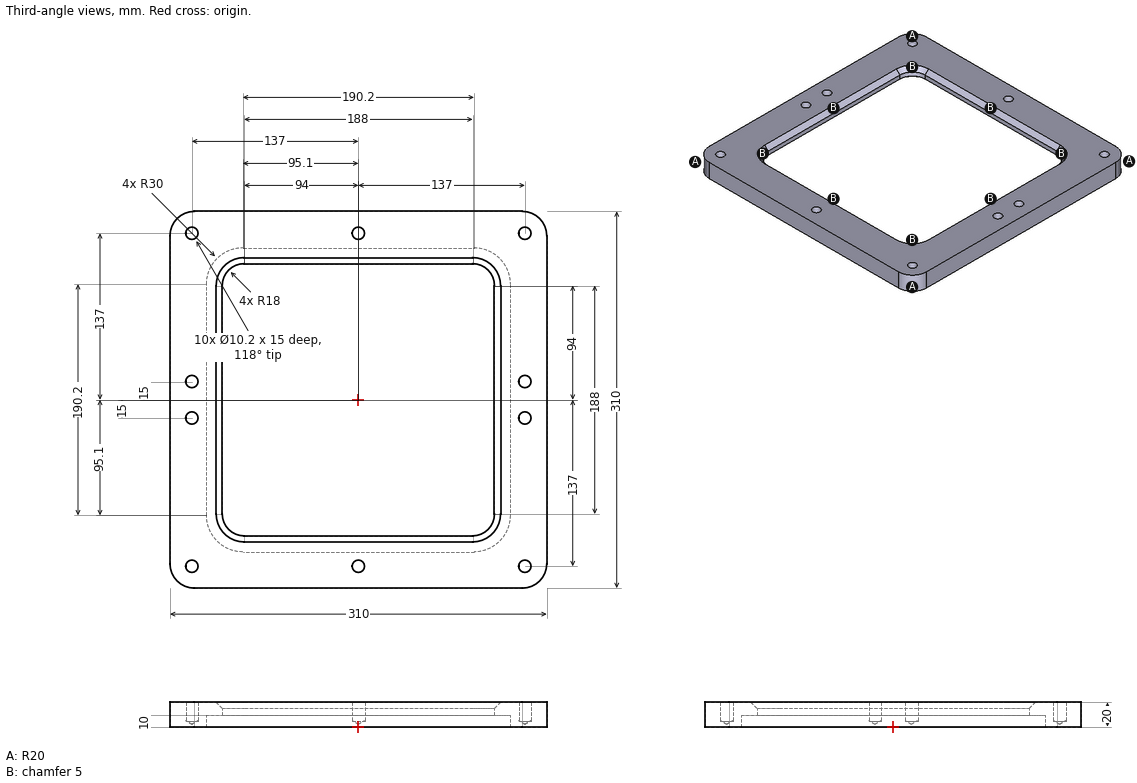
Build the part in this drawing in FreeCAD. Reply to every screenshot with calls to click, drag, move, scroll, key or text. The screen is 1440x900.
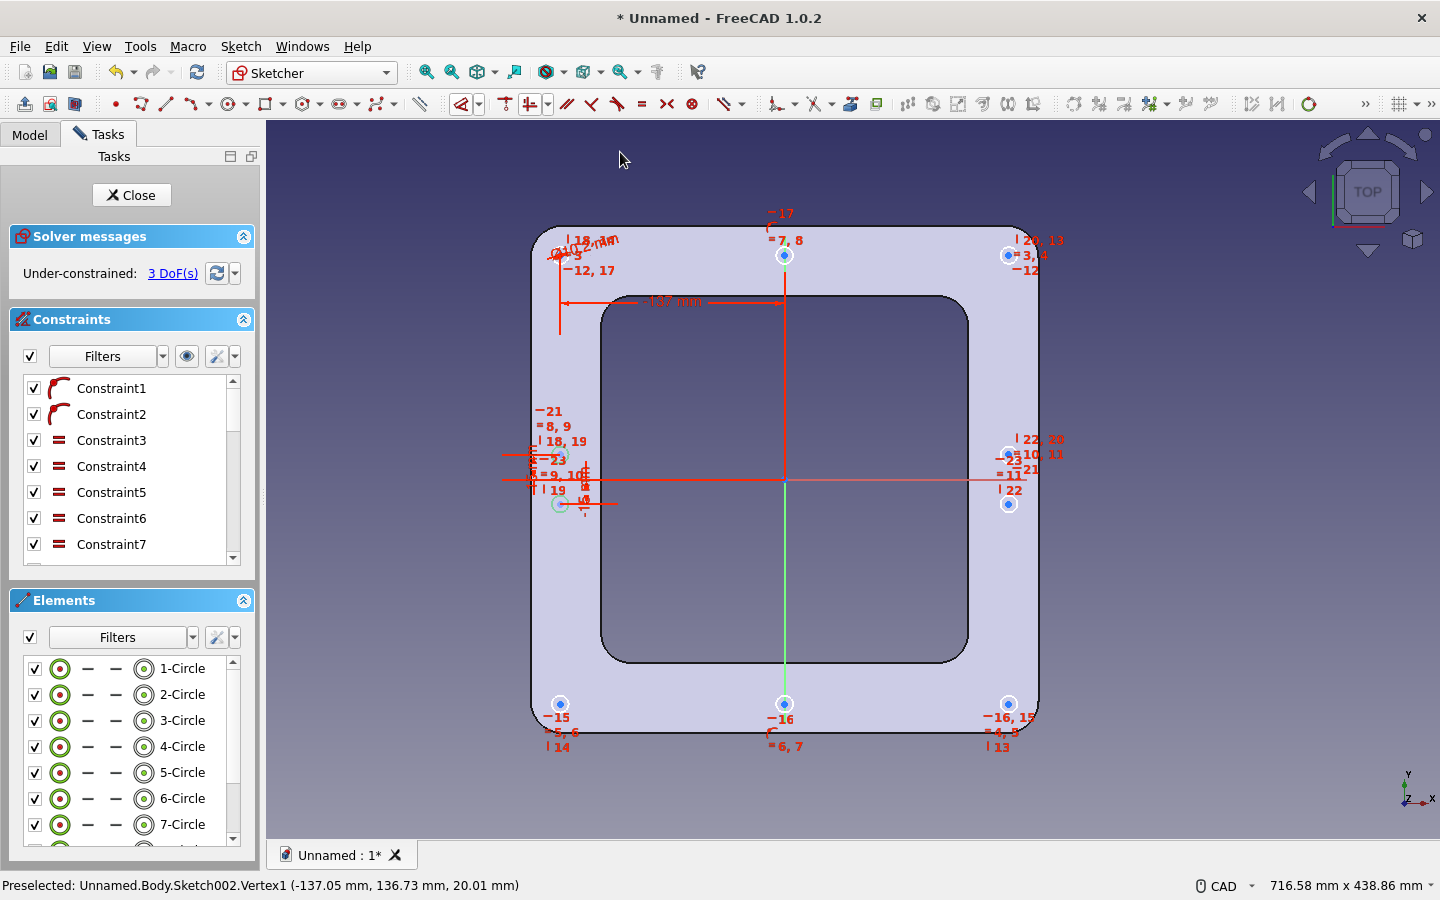
click(560, 255)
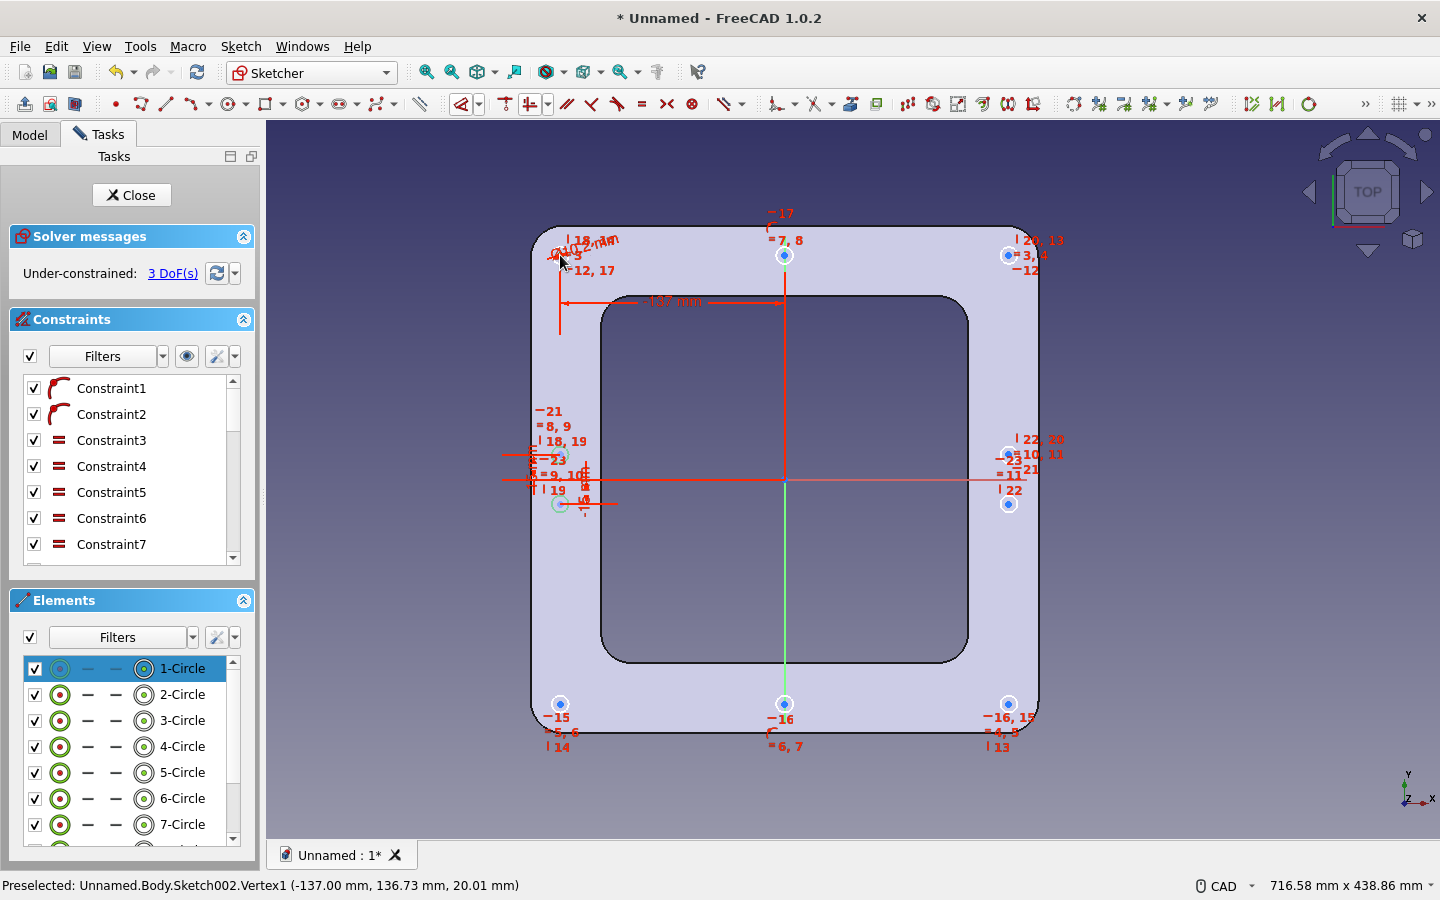
click(478, 104)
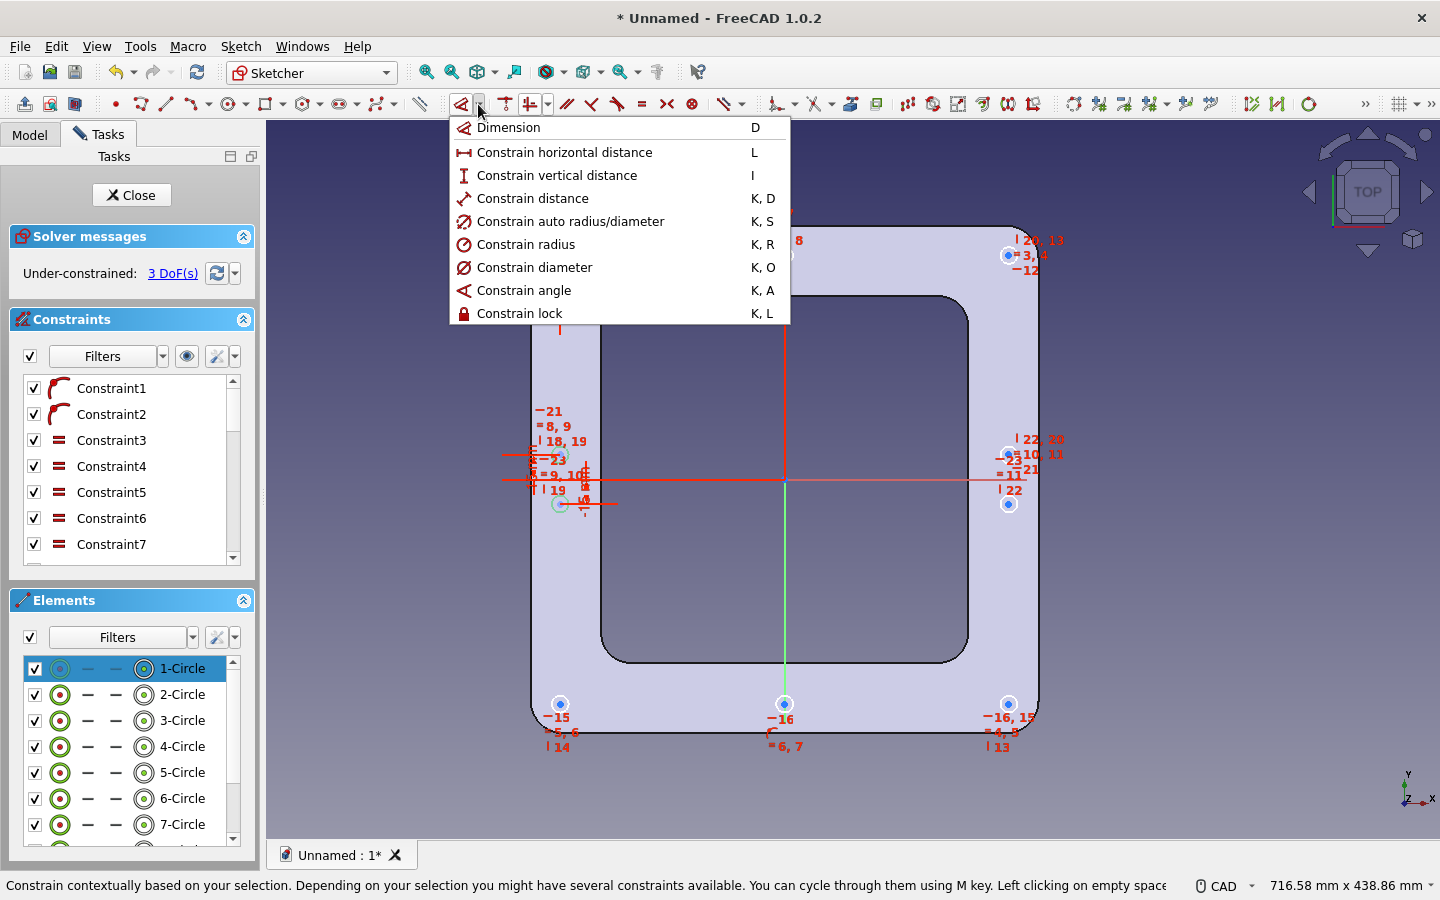
click(620, 176)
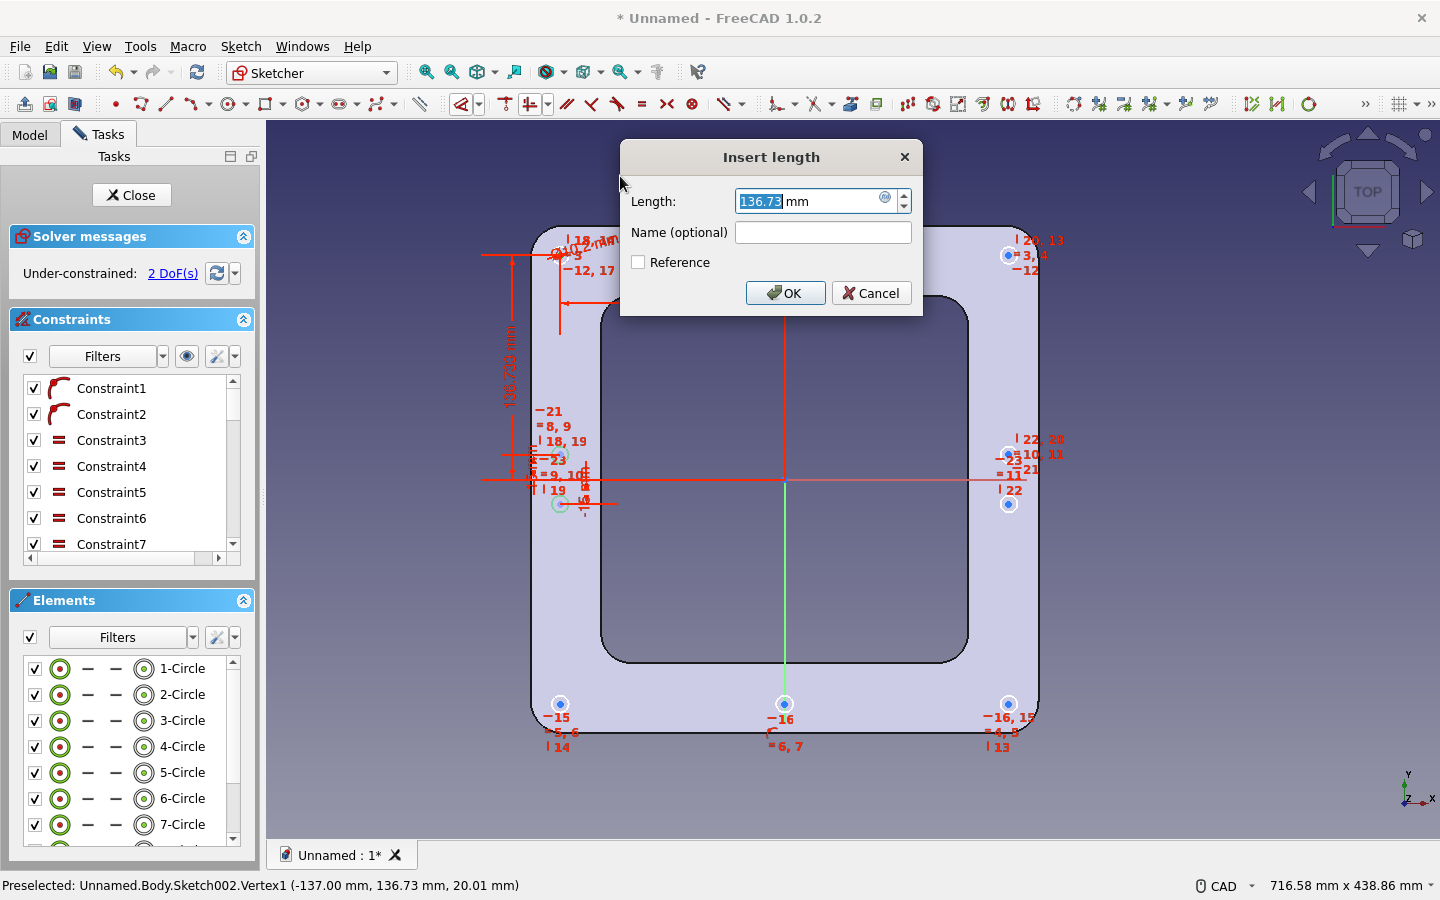
text(137)
key(Return)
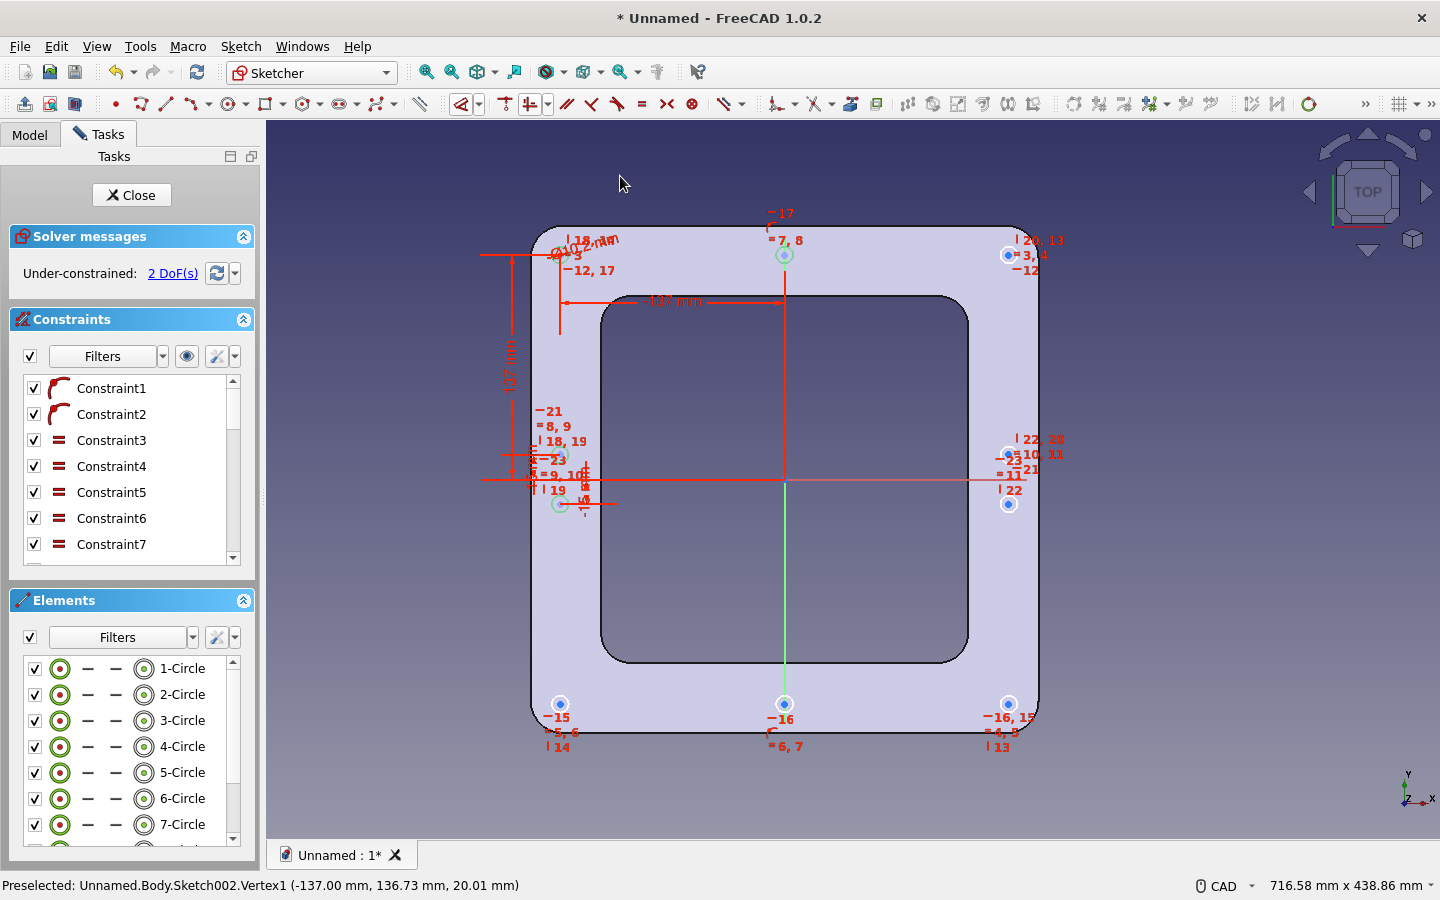
click(1009, 255)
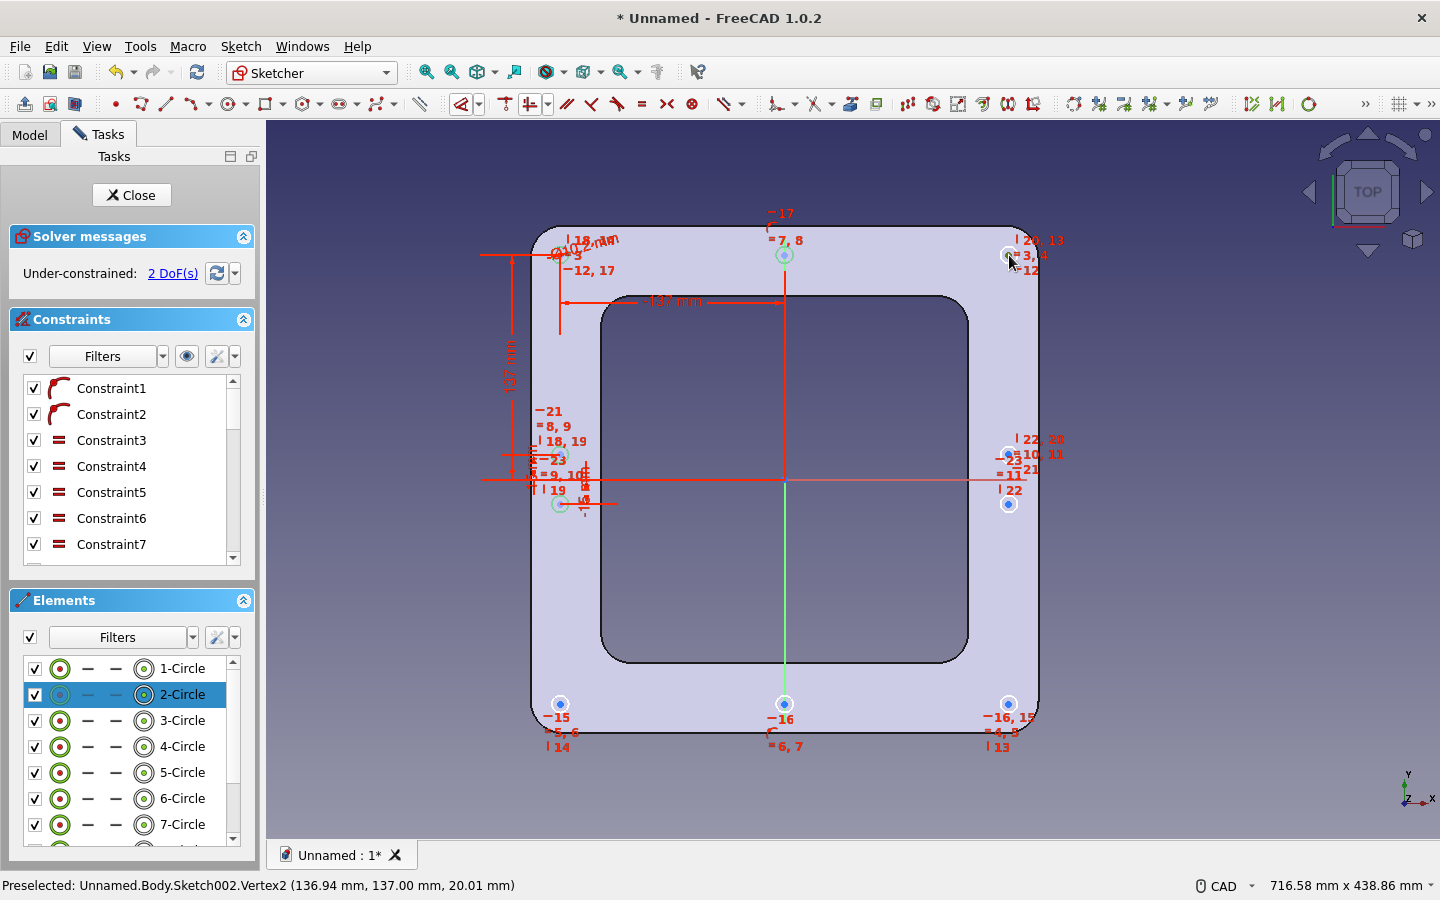
click(478, 104)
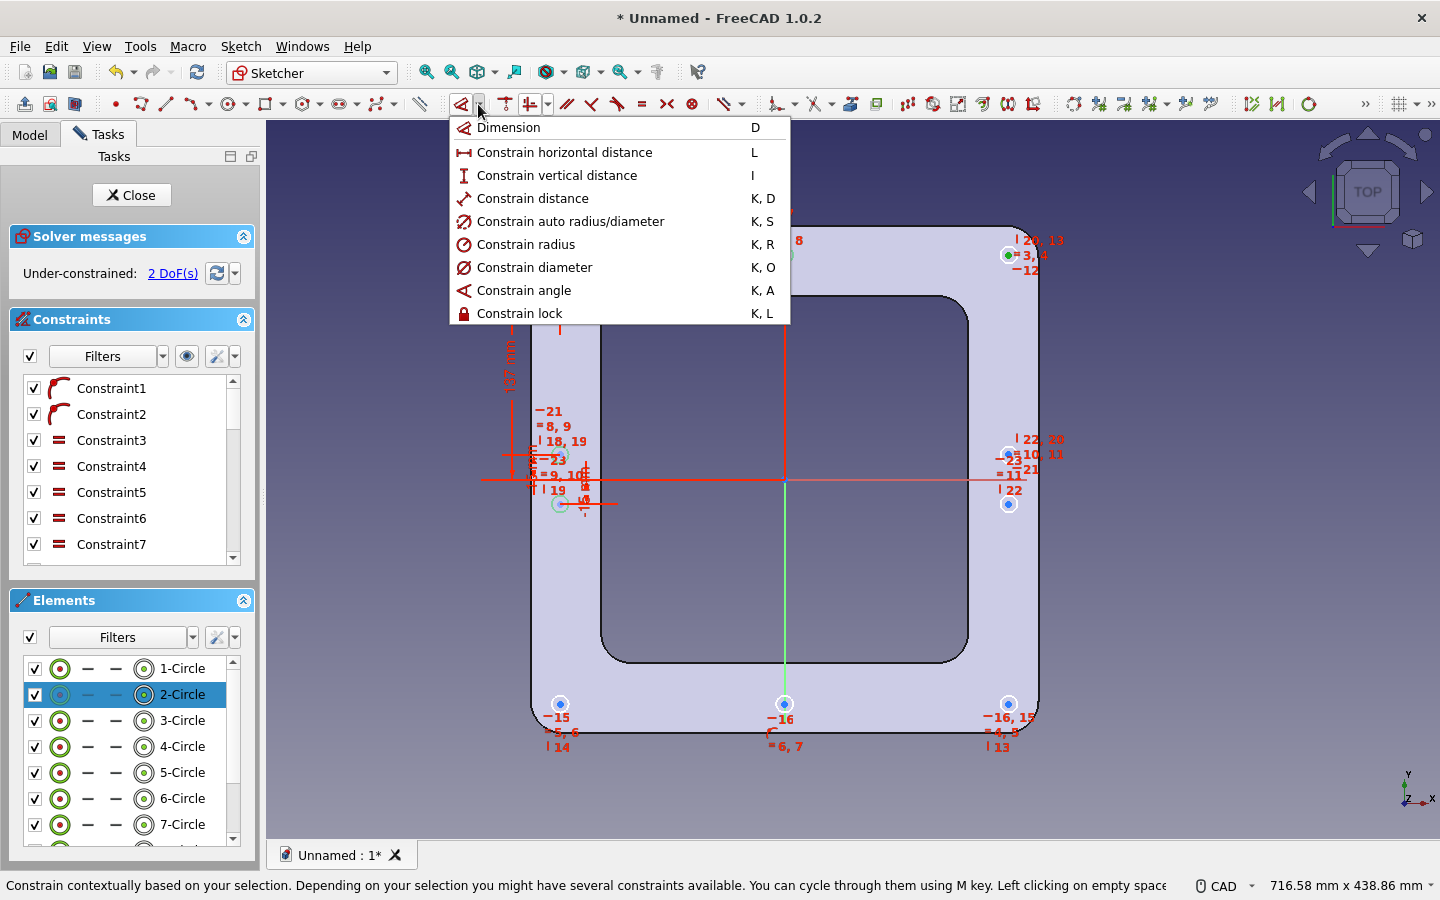
click(620, 152)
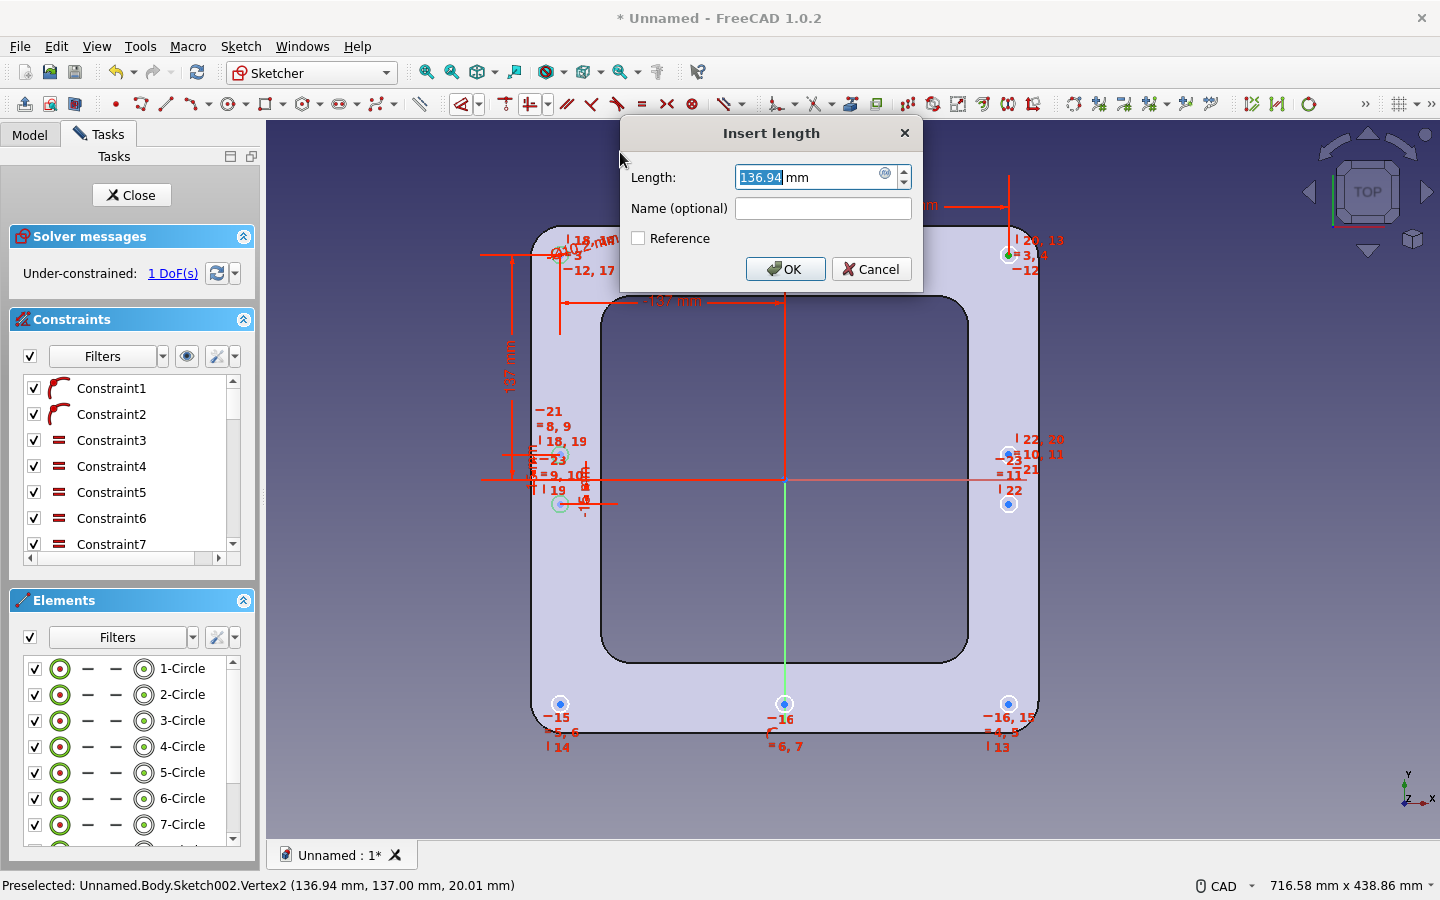
text(137)
key(Return)